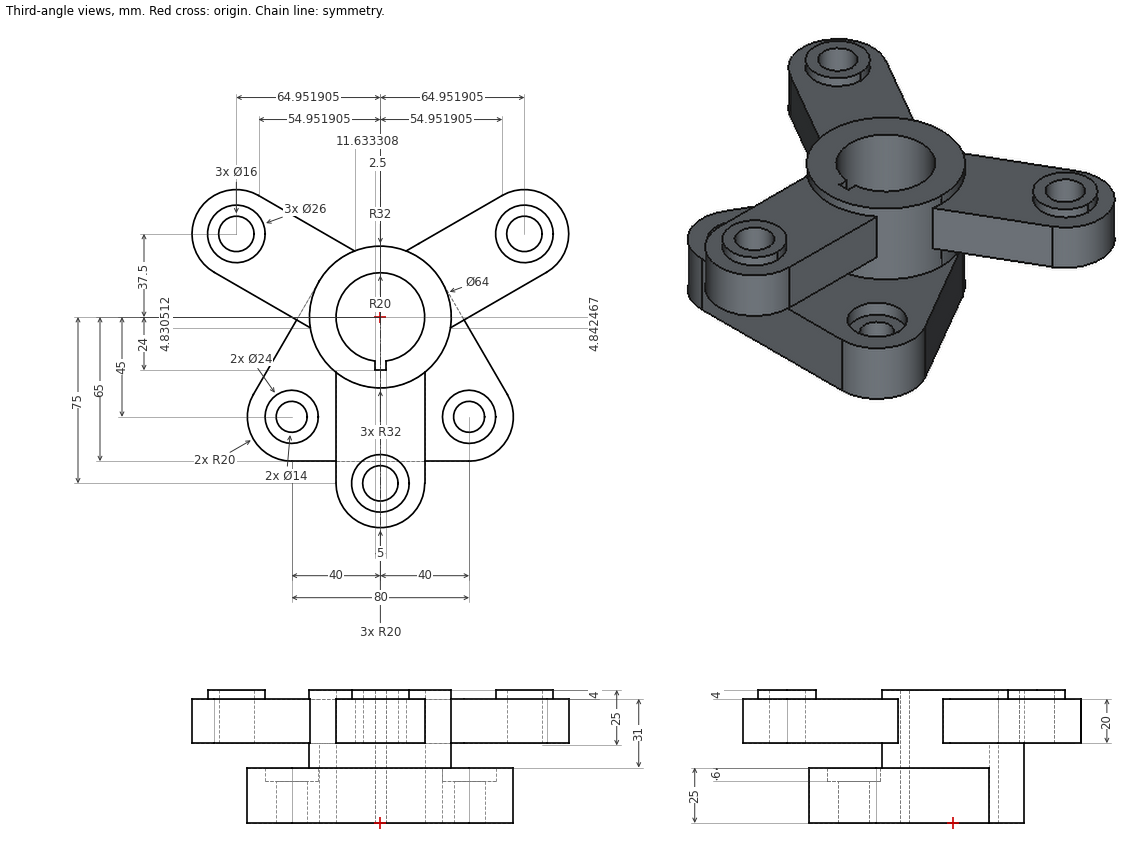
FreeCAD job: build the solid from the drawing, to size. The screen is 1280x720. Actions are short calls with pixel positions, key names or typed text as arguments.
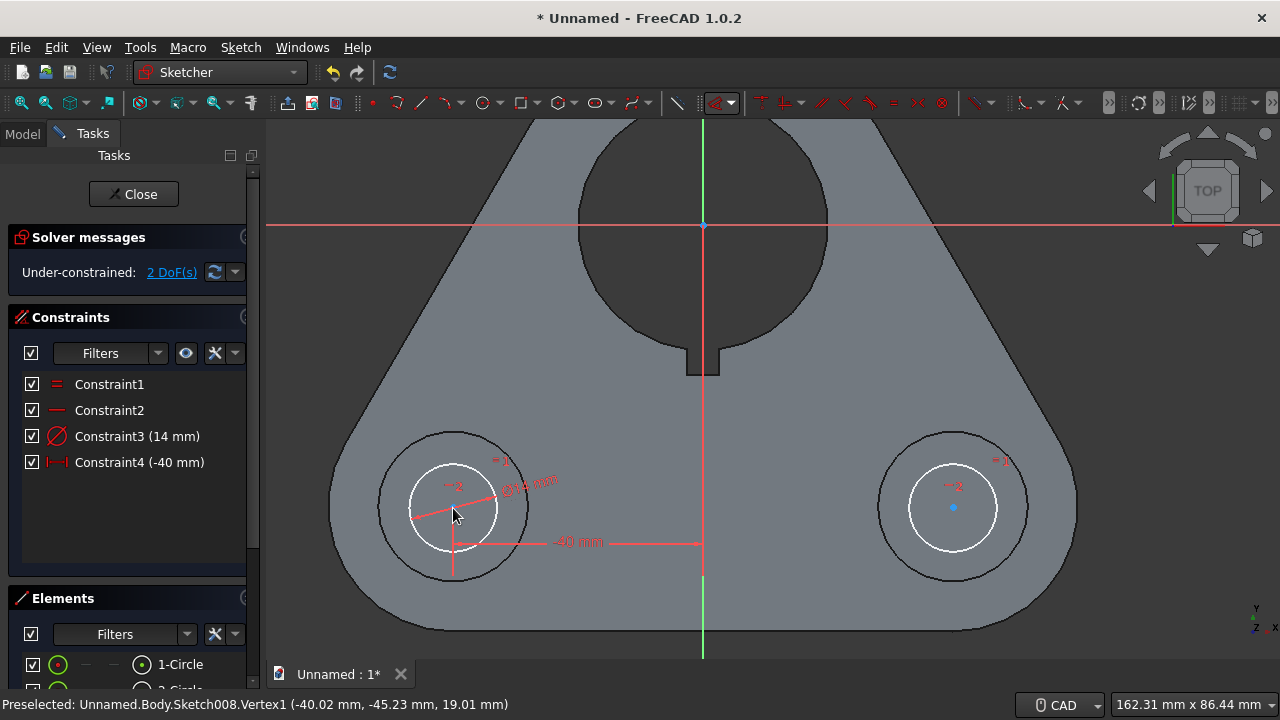
click(453, 508)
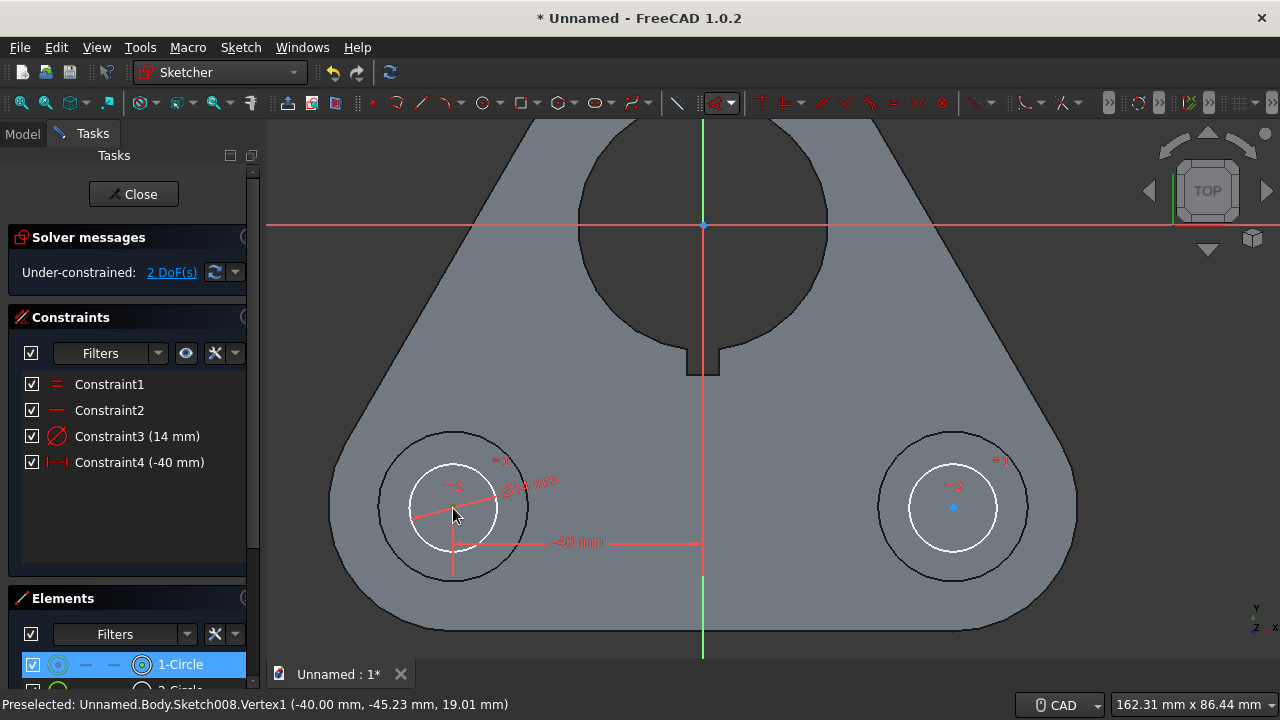
key(i)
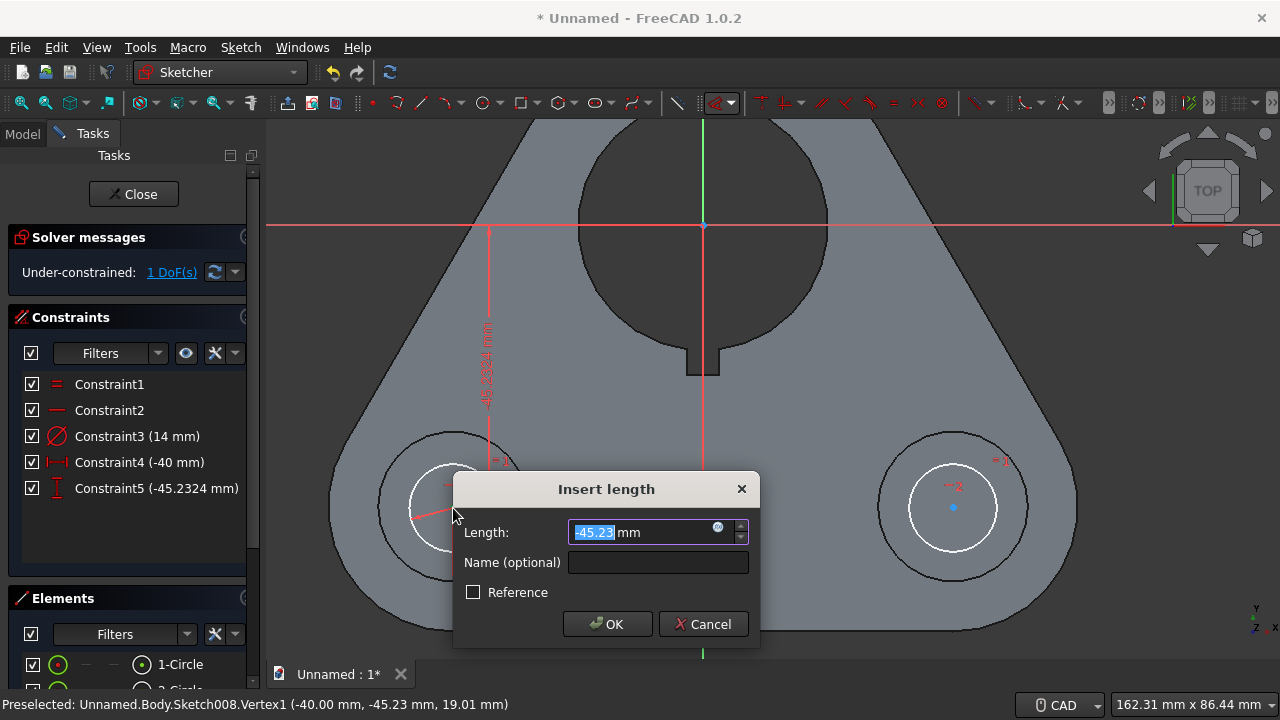
text(-45)
key(Return)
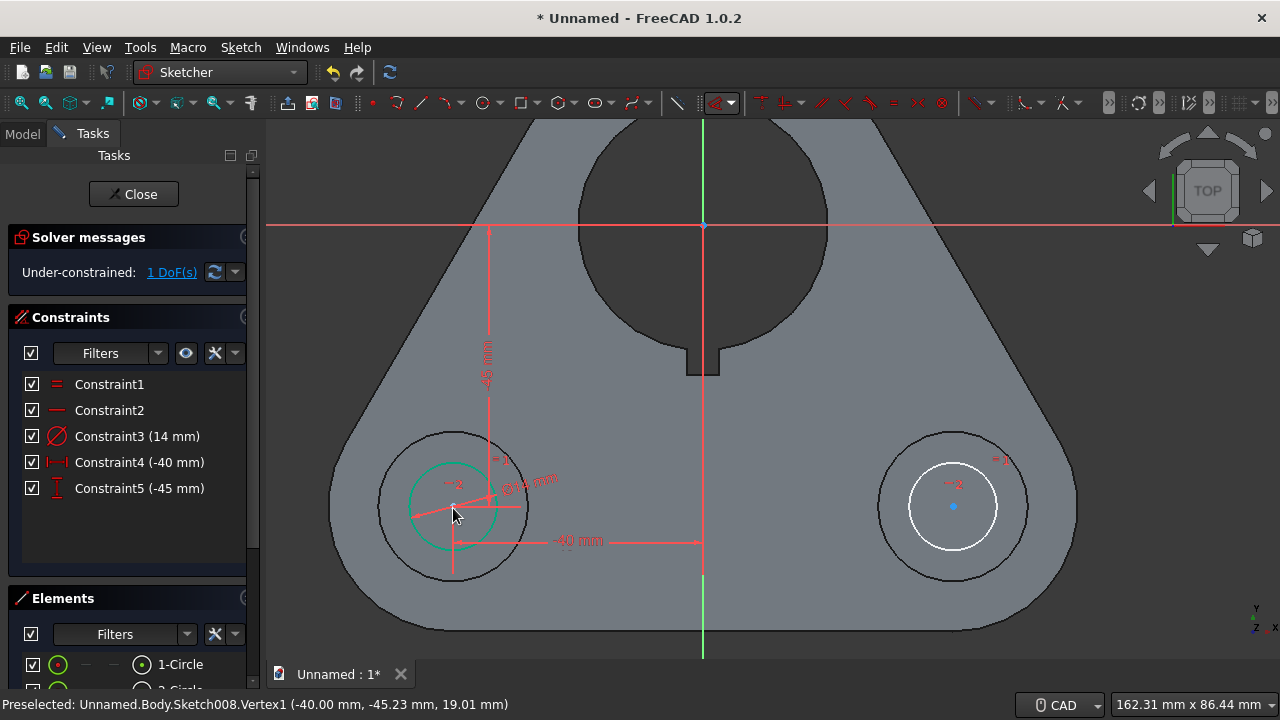
click(953, 507)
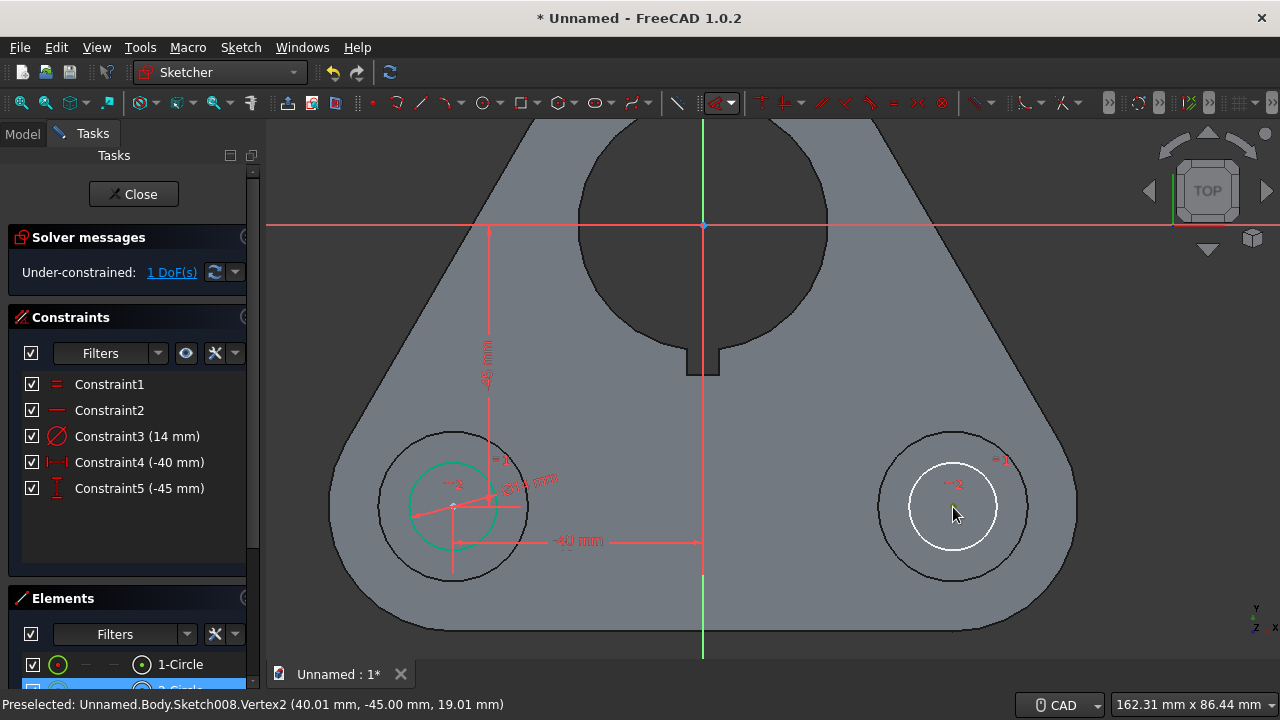
key(l)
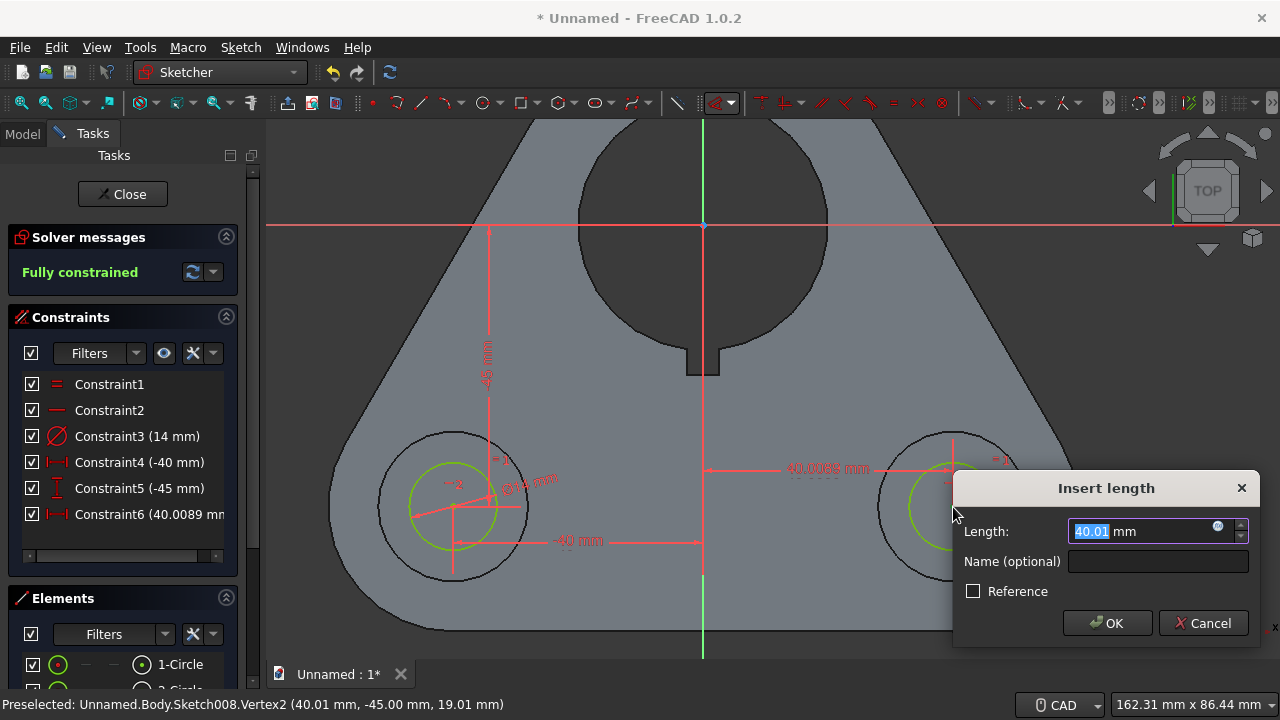
text(40)
key(Return)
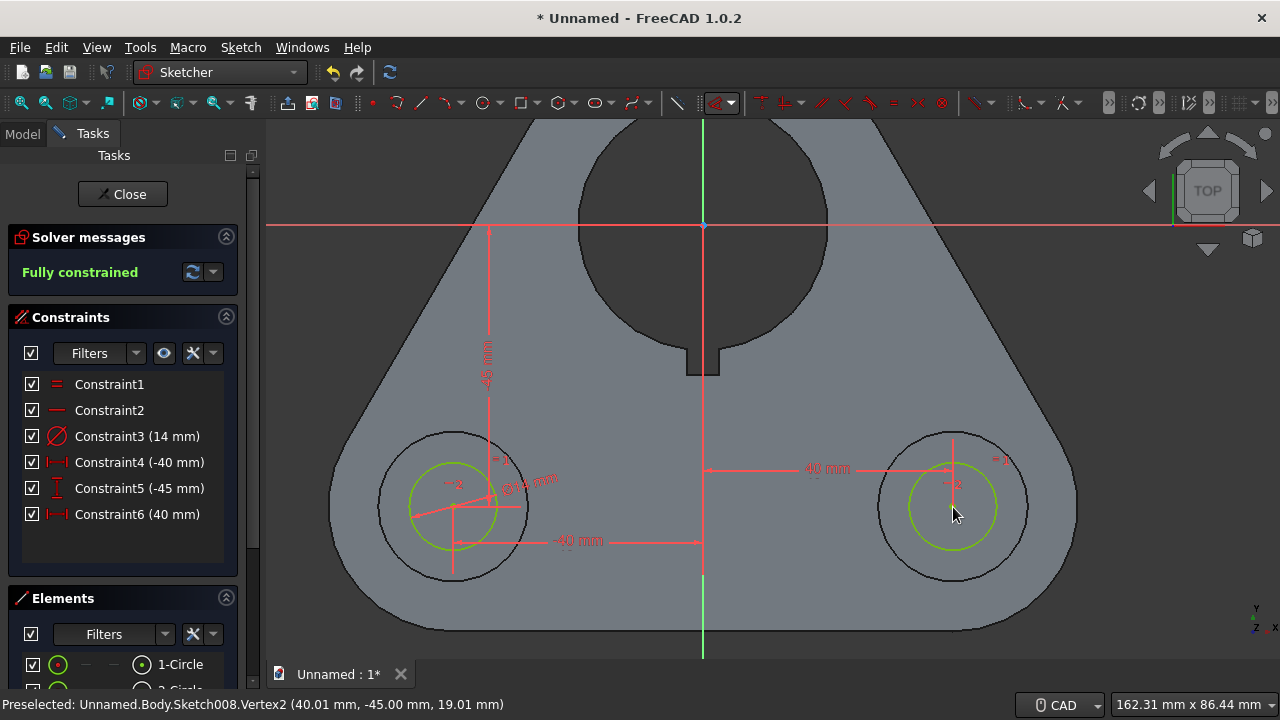
click(123, 194)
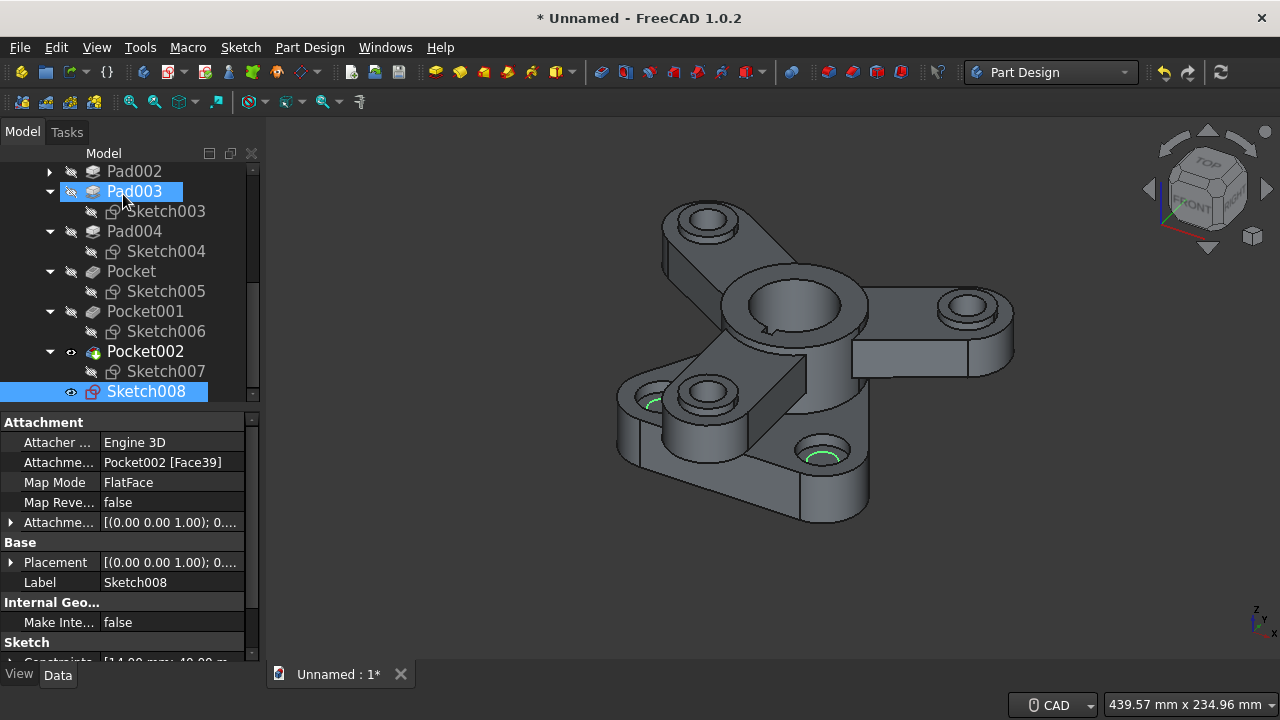
click(602, 72)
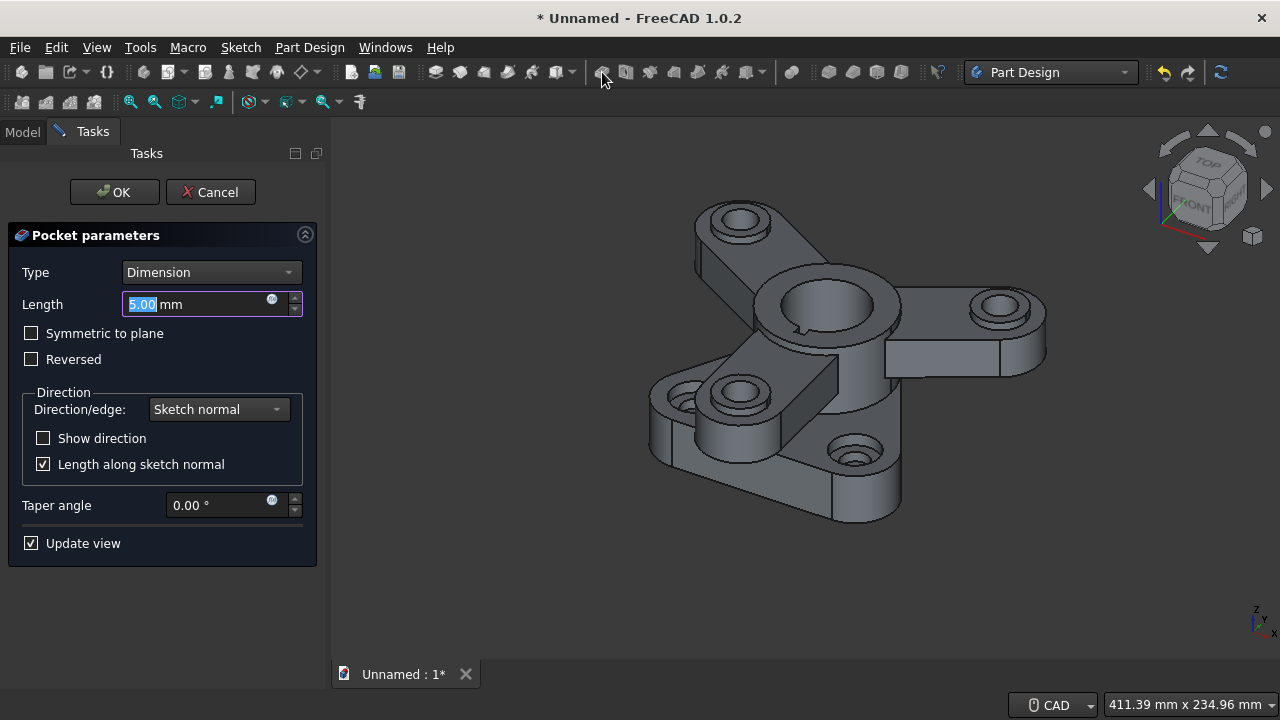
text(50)
key(Tab)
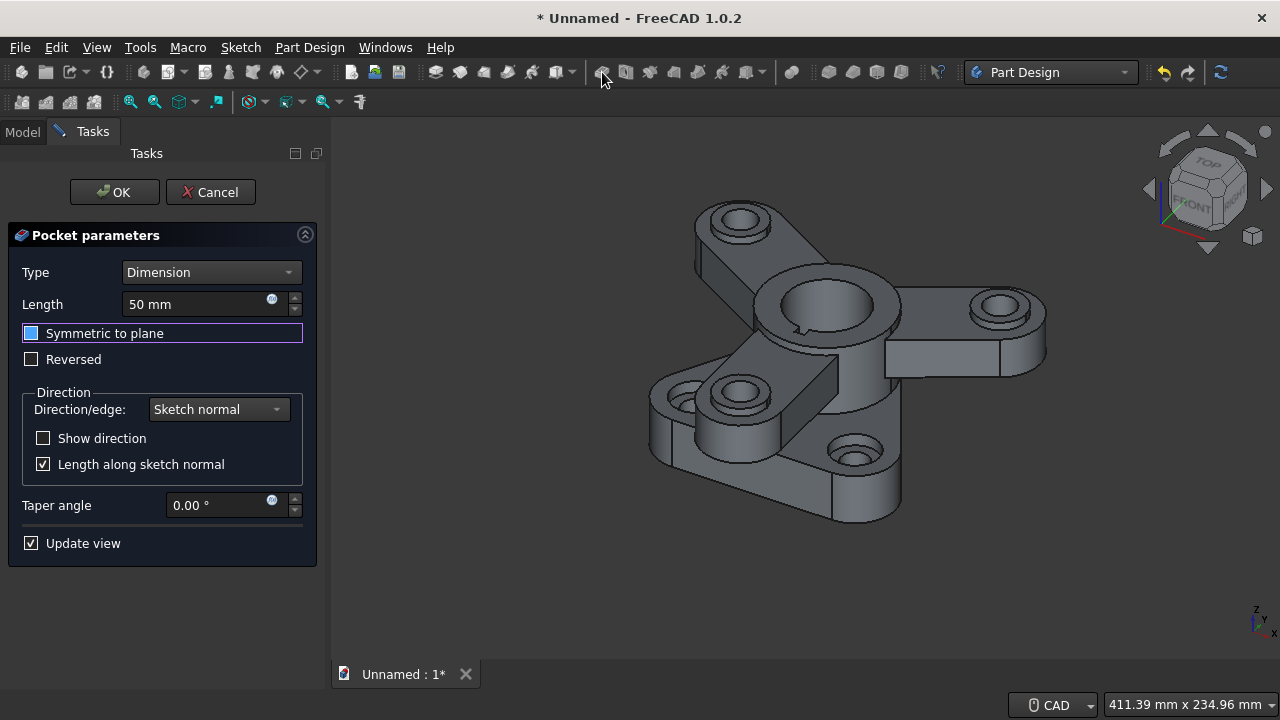
click(115, 192)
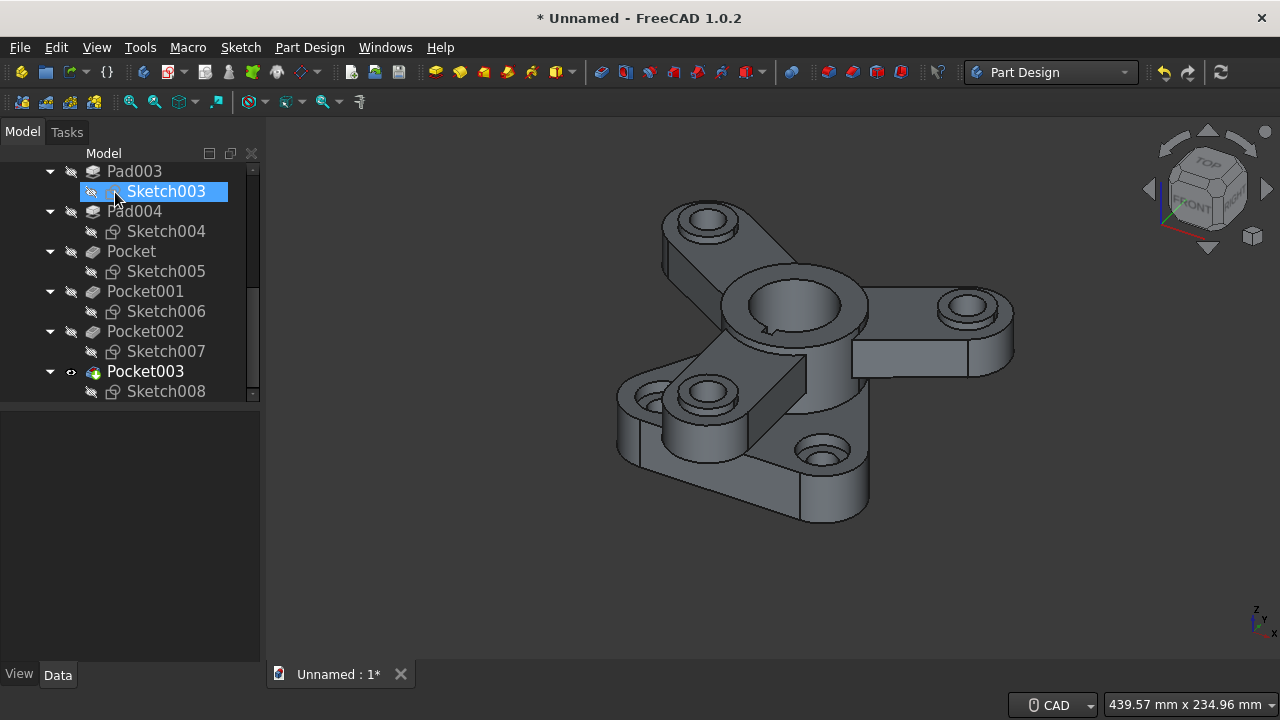
key(0)